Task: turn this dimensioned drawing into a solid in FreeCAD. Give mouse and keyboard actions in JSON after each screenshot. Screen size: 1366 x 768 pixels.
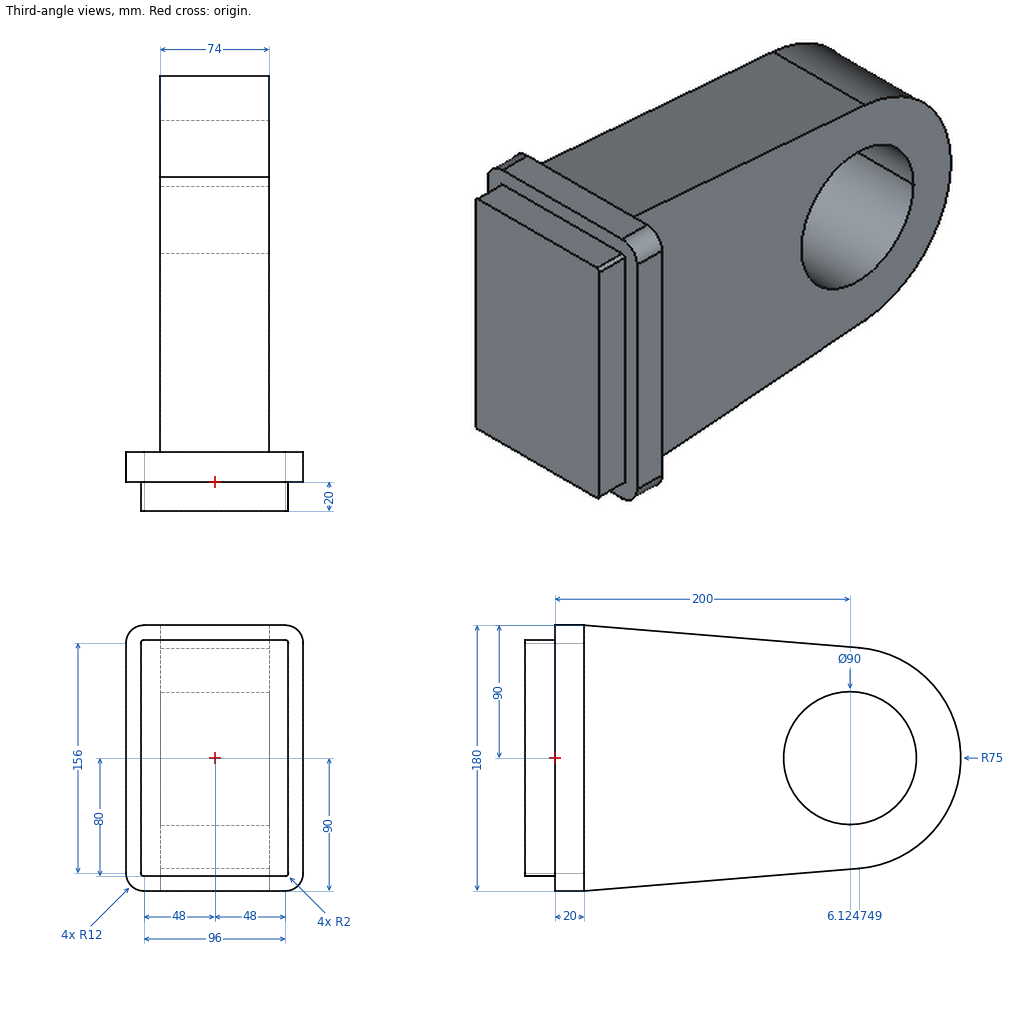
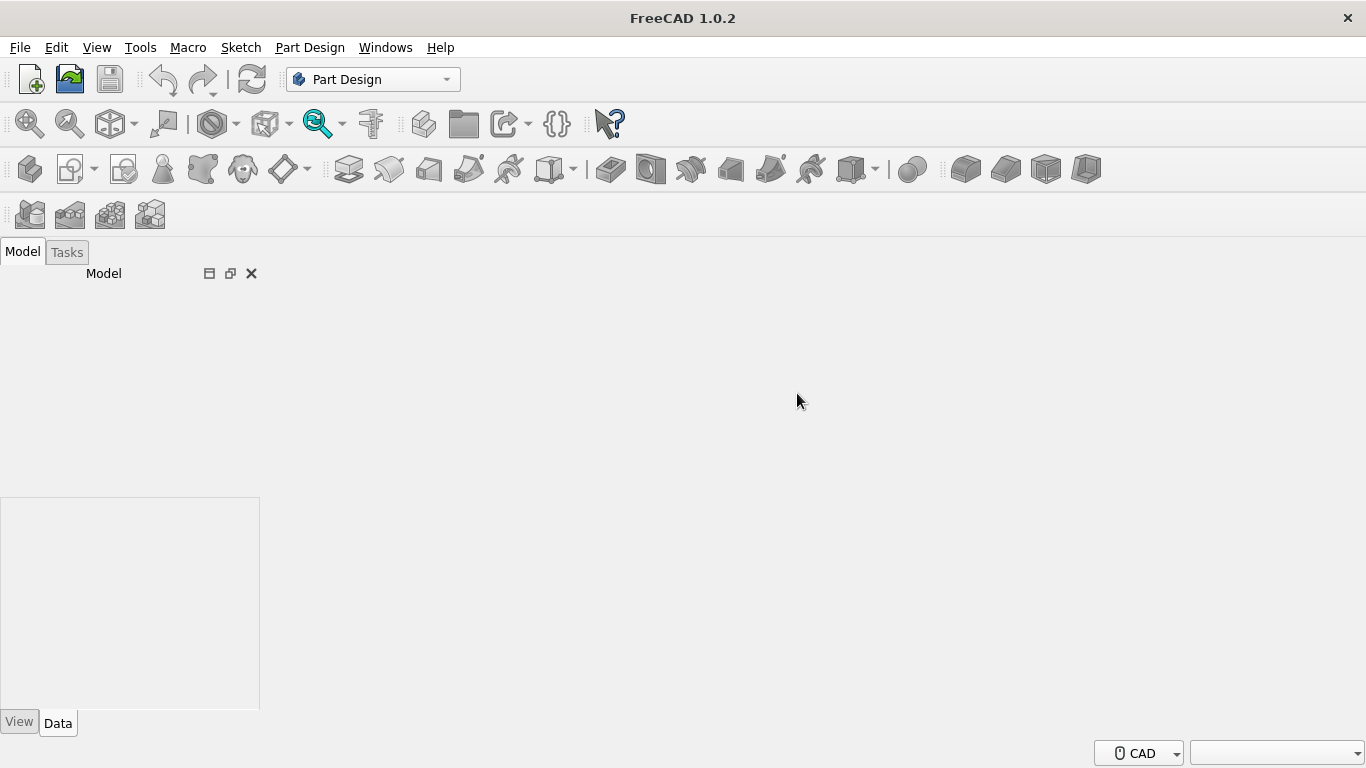
{"action": "key", "text": "ctrl+n"}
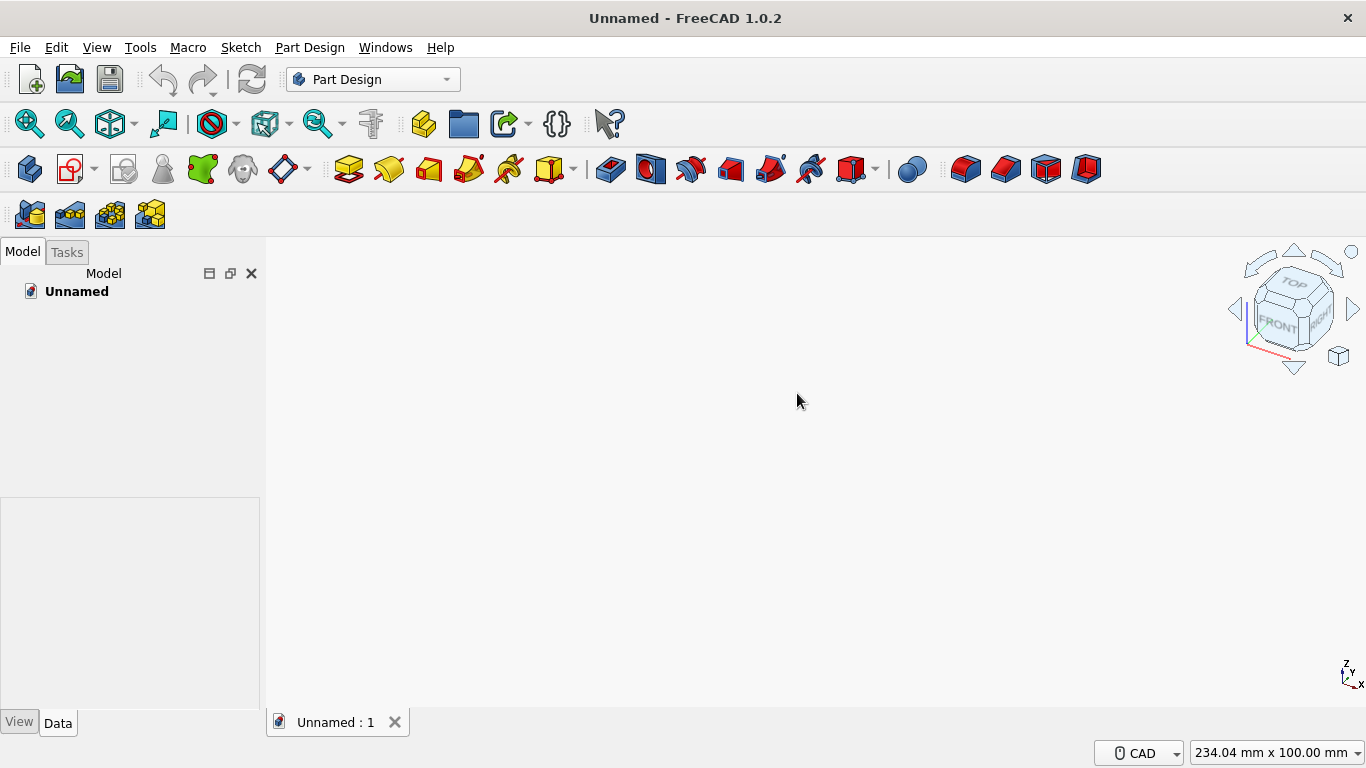
{"action": "left_click", "coordinate": [70, 170]}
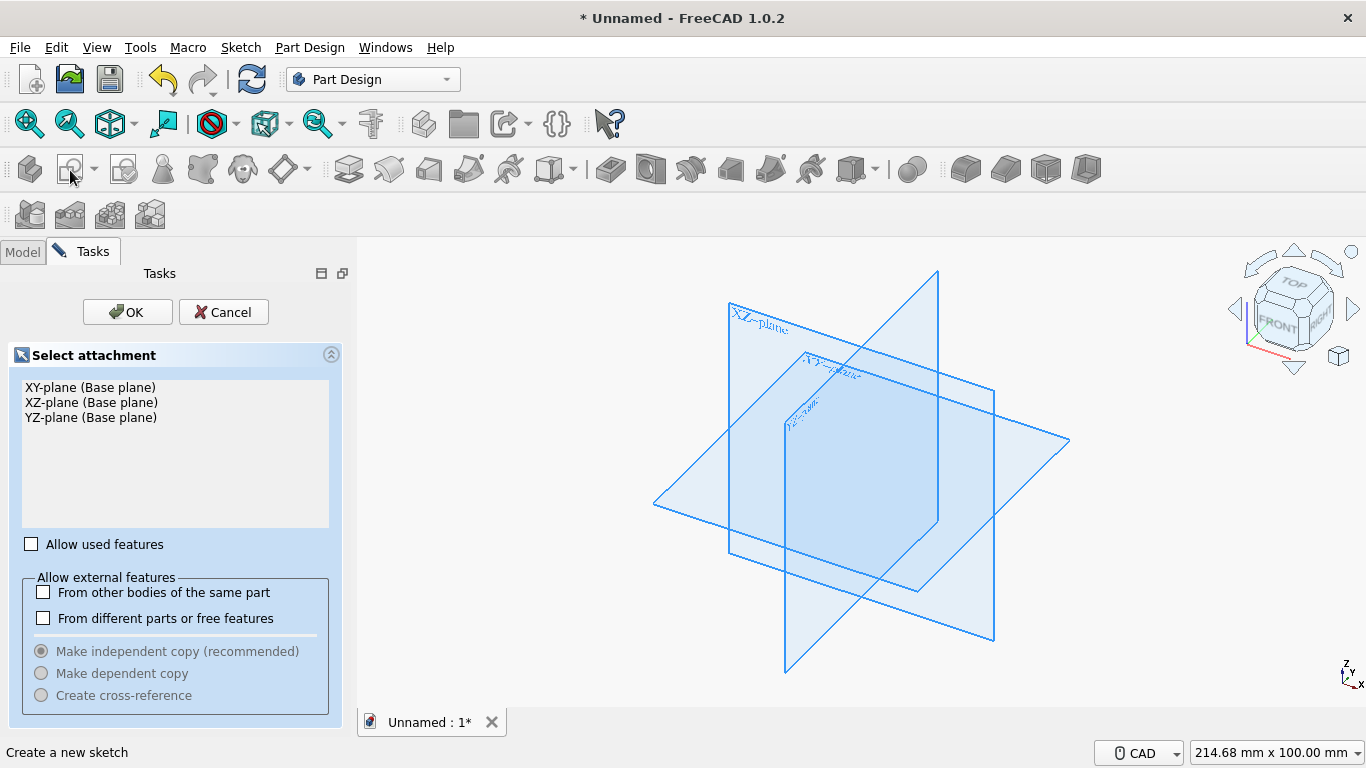
{"action": "left_click", "coordinate": [82, 402]}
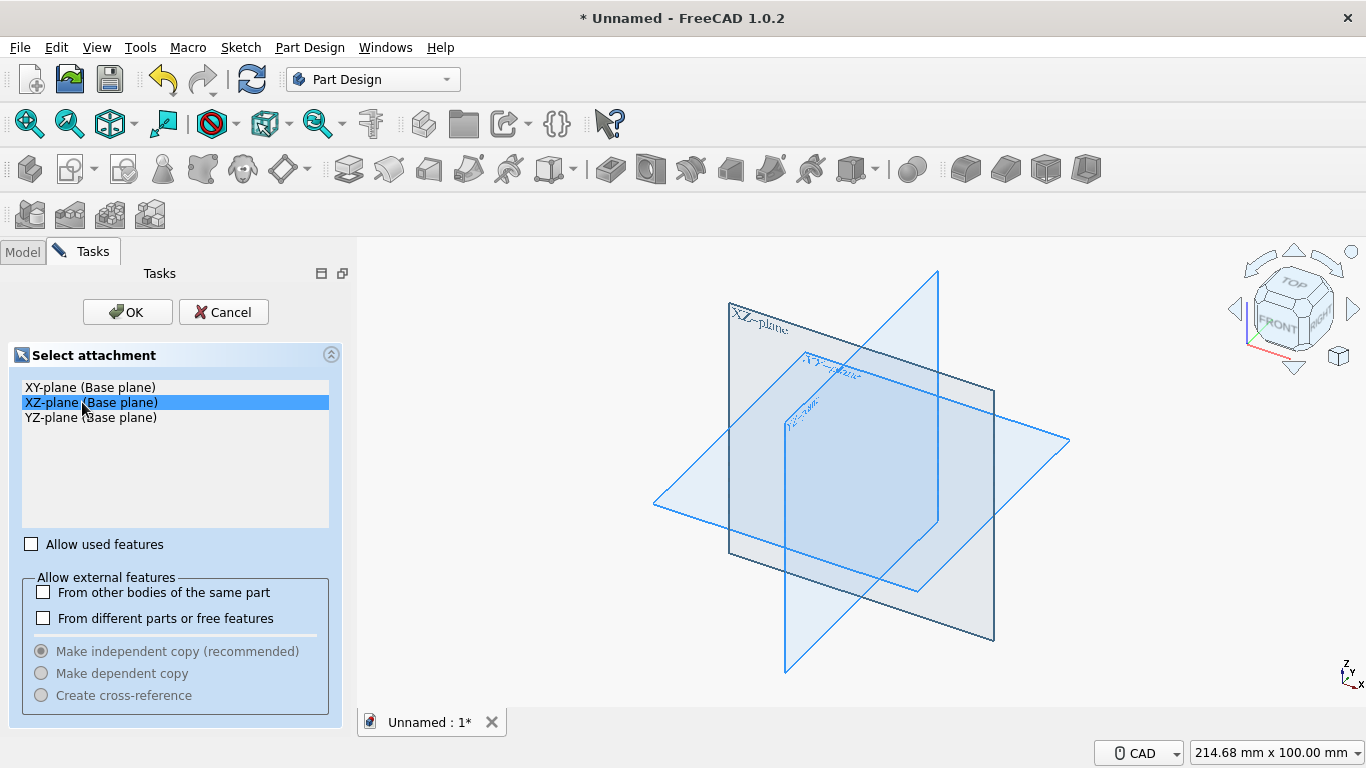
{"action": "left_click", "coordinate": [128, 312]}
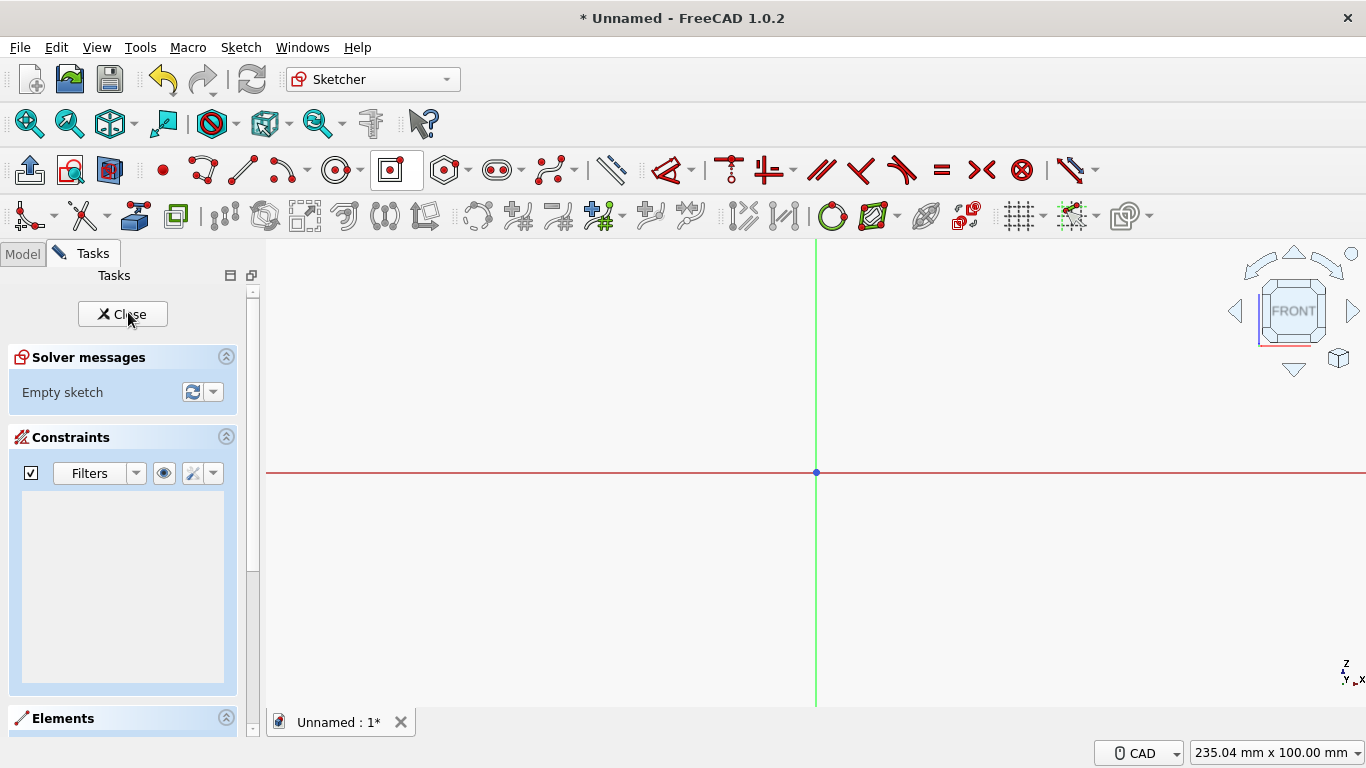
{"action": "scroll", "coordinate": [708, 473], "scroll_direction": "down", "scroll_amount": 5}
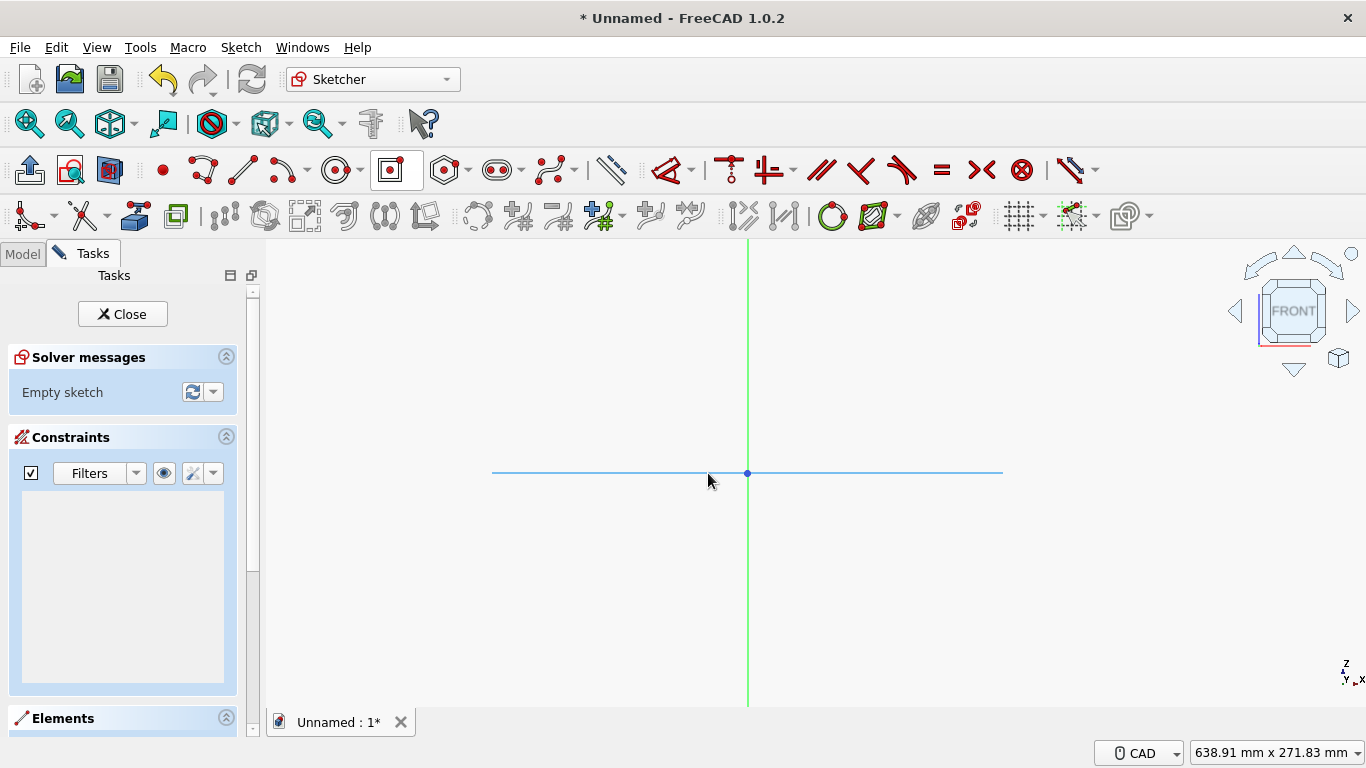
{"action": "key", "text": "g l"}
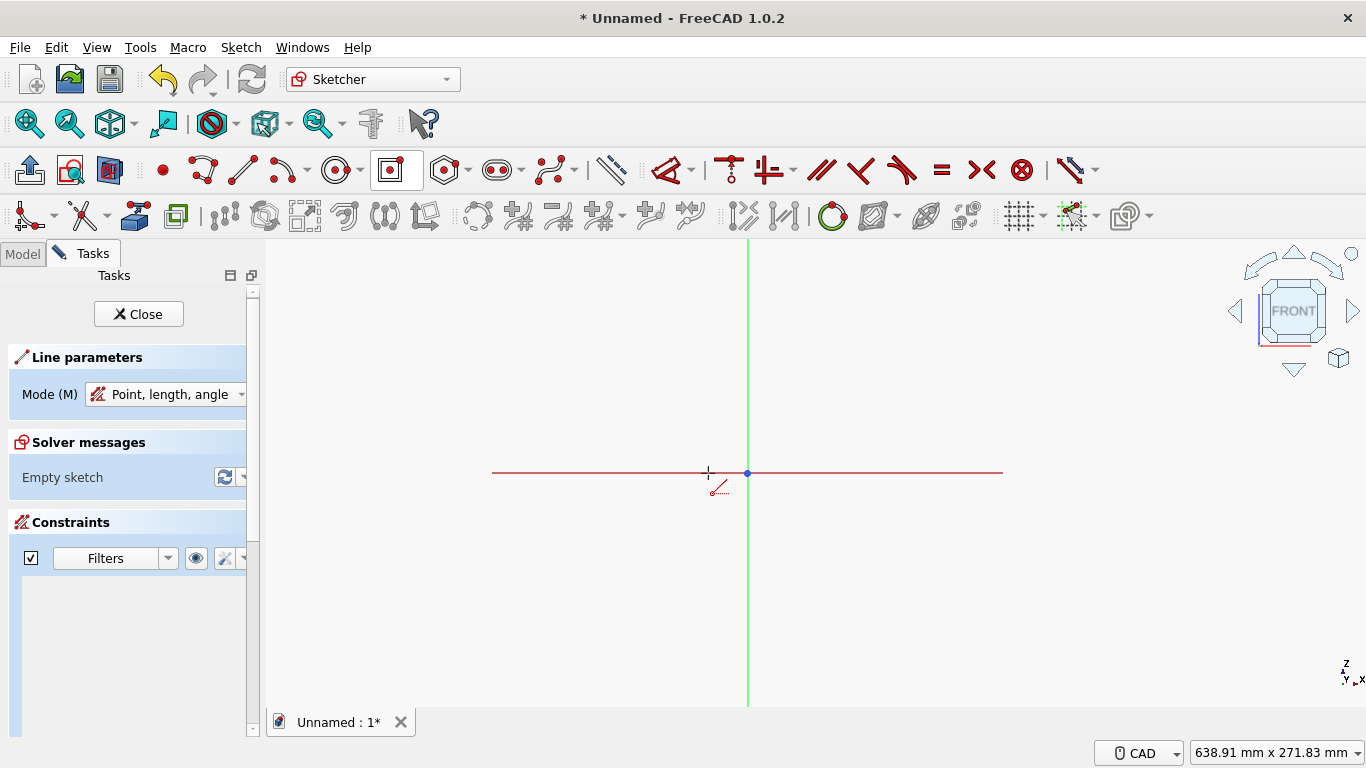
{"action": "left_click", "coordinate": [831, 628]}
{"action": "left_click", "coordinate": [665, 628]}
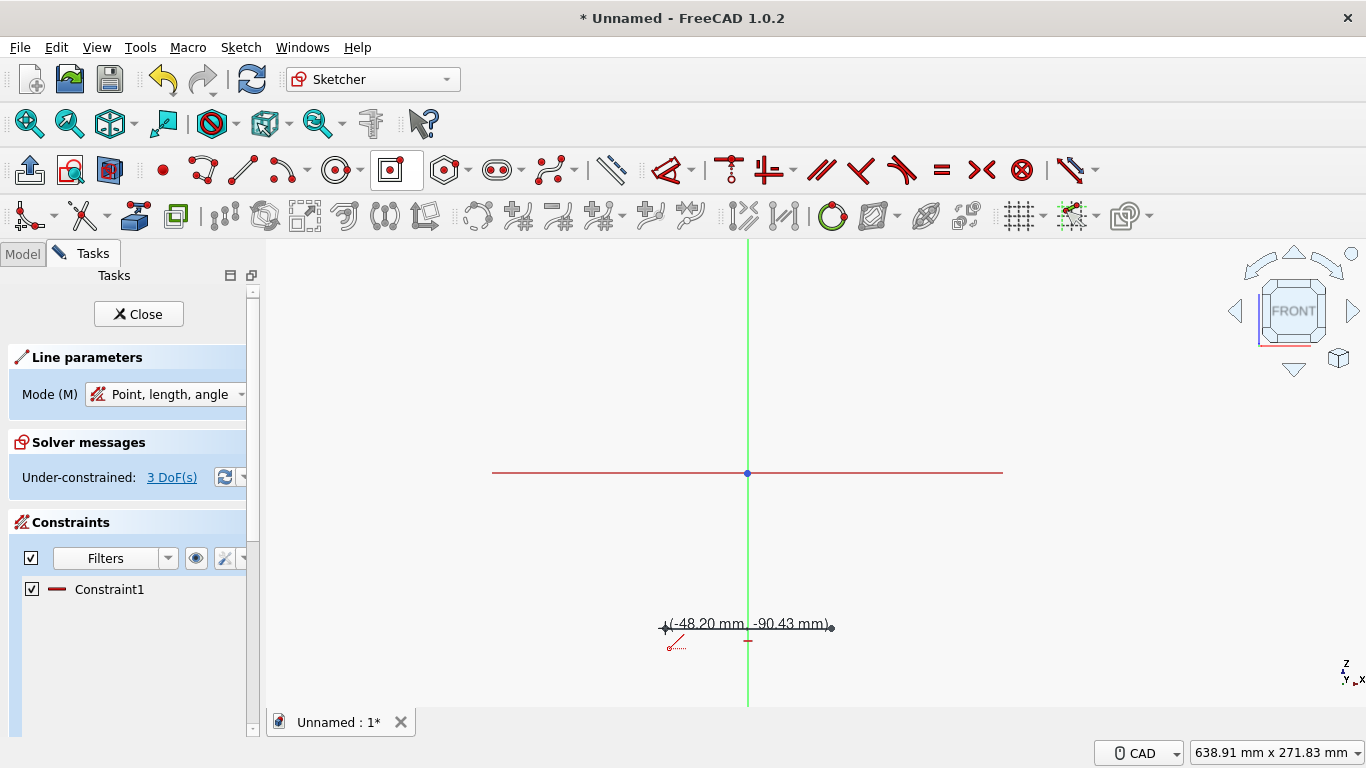
{"action": "left_click", "coordinate": [645, 608]}
{"action": "left_click", "coordinate": [645, 339]}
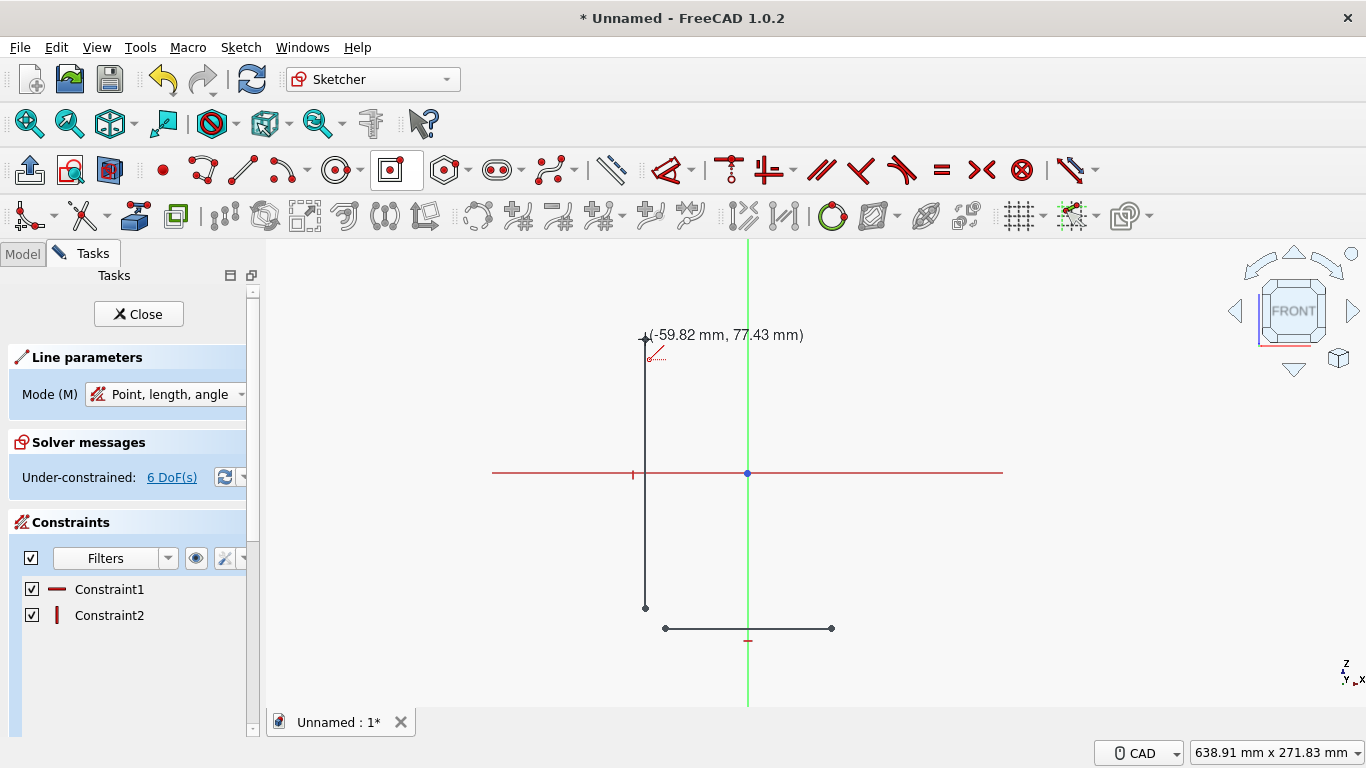
{"action": "left_click", "coordinate": [665, 318]}
{"action": "left_click", "coordinate": [831, 318]}